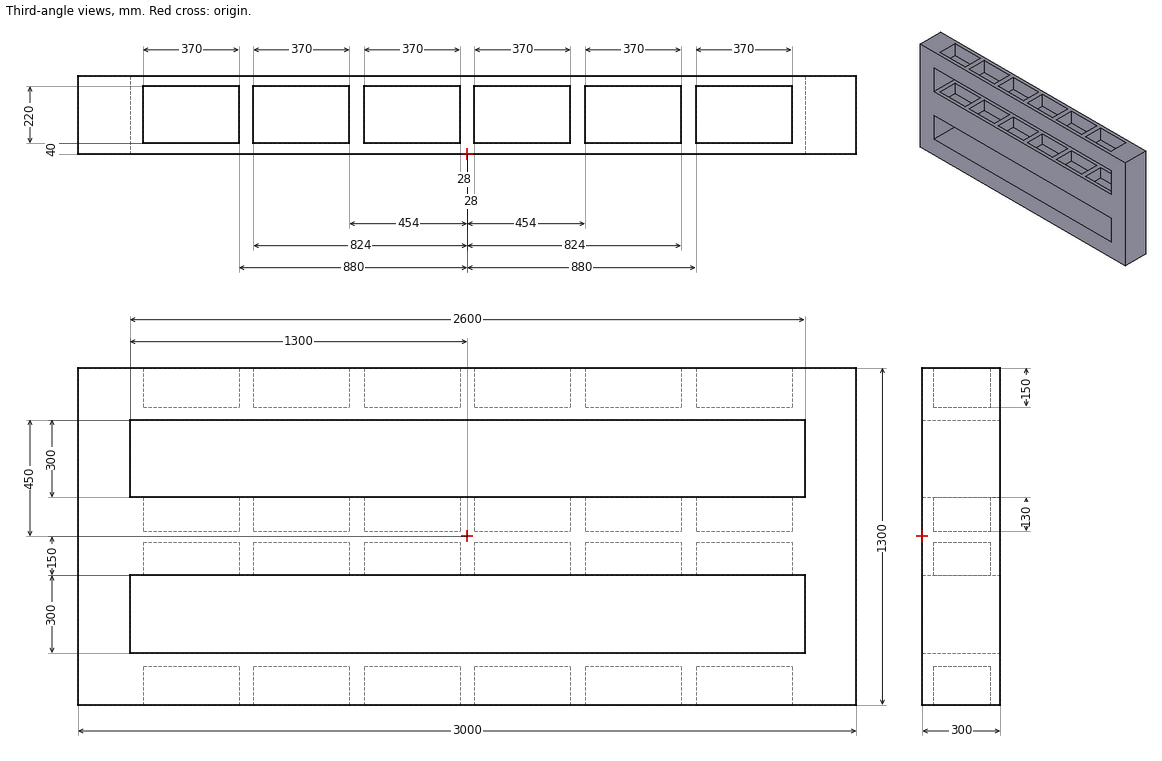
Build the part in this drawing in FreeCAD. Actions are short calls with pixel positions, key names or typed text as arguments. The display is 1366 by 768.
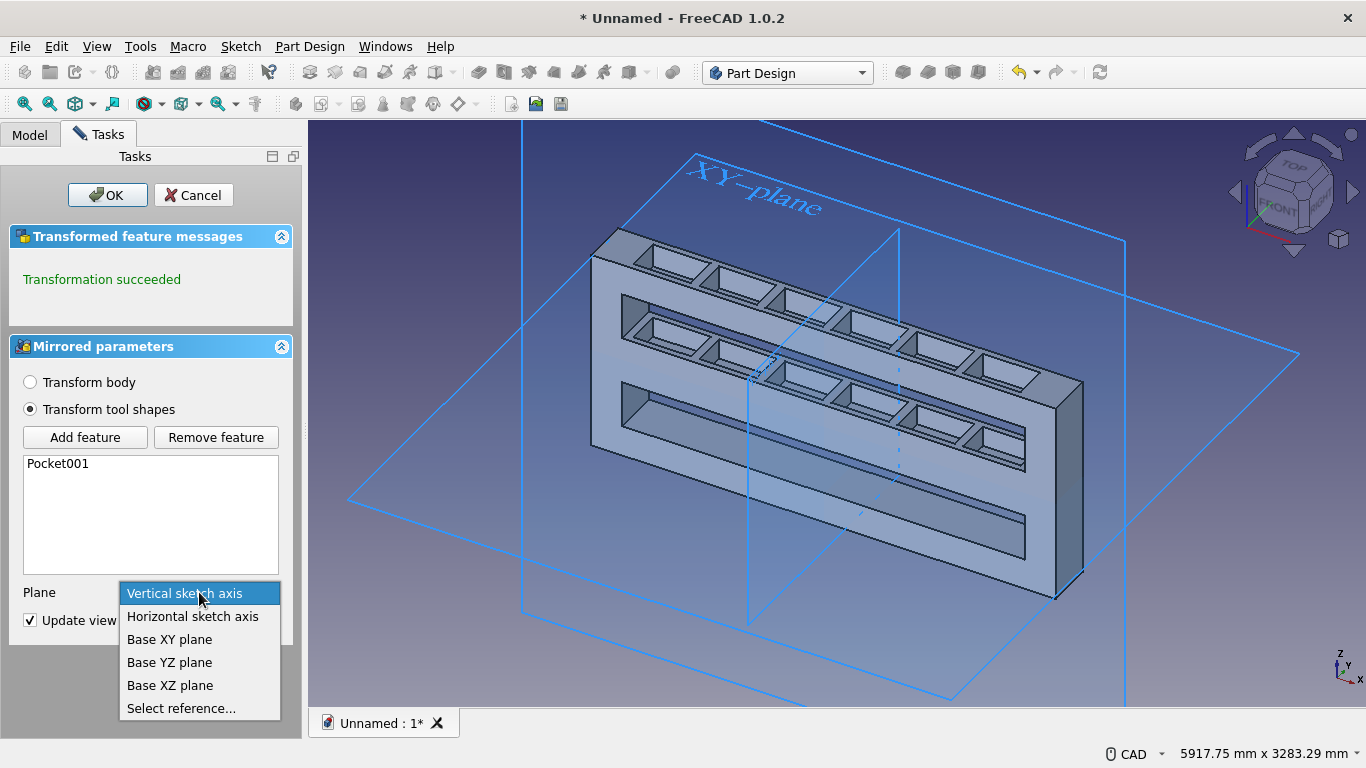
click(198, 640)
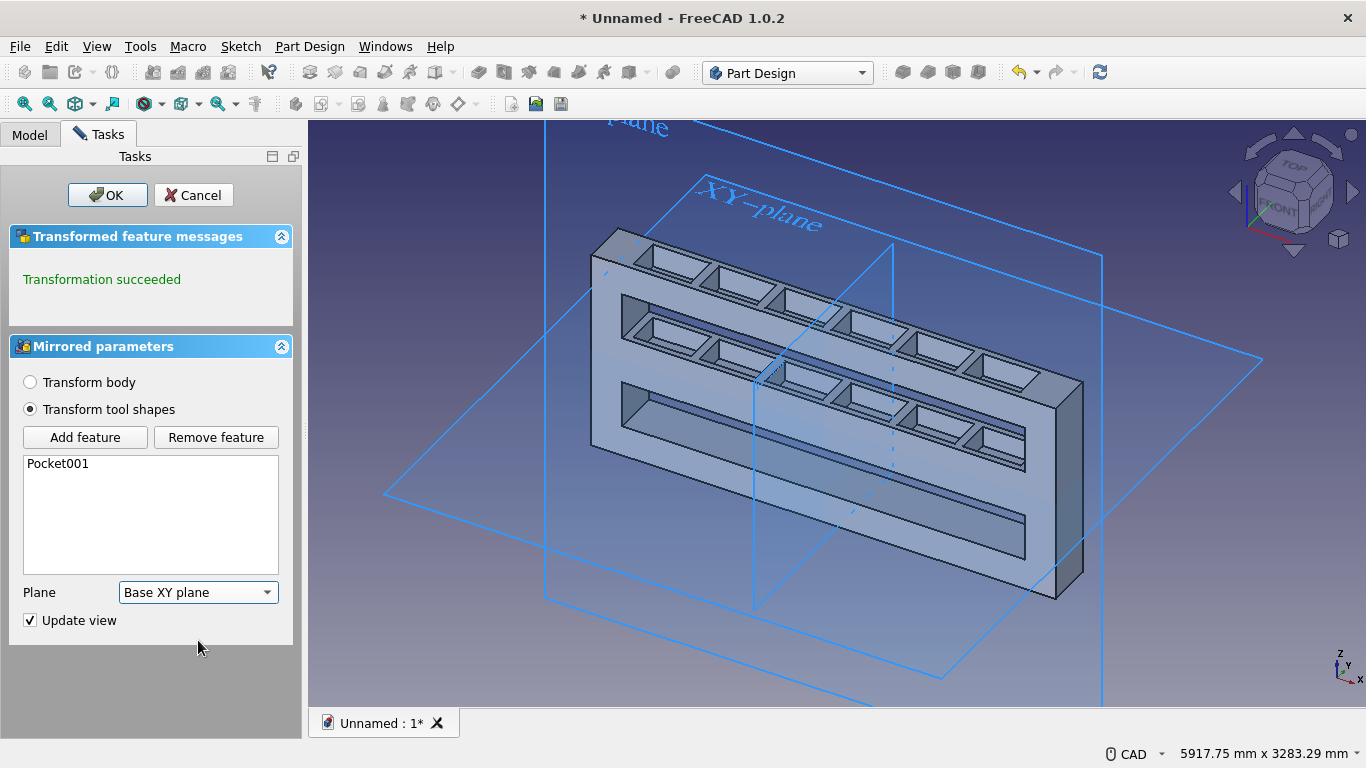
click(108, 195)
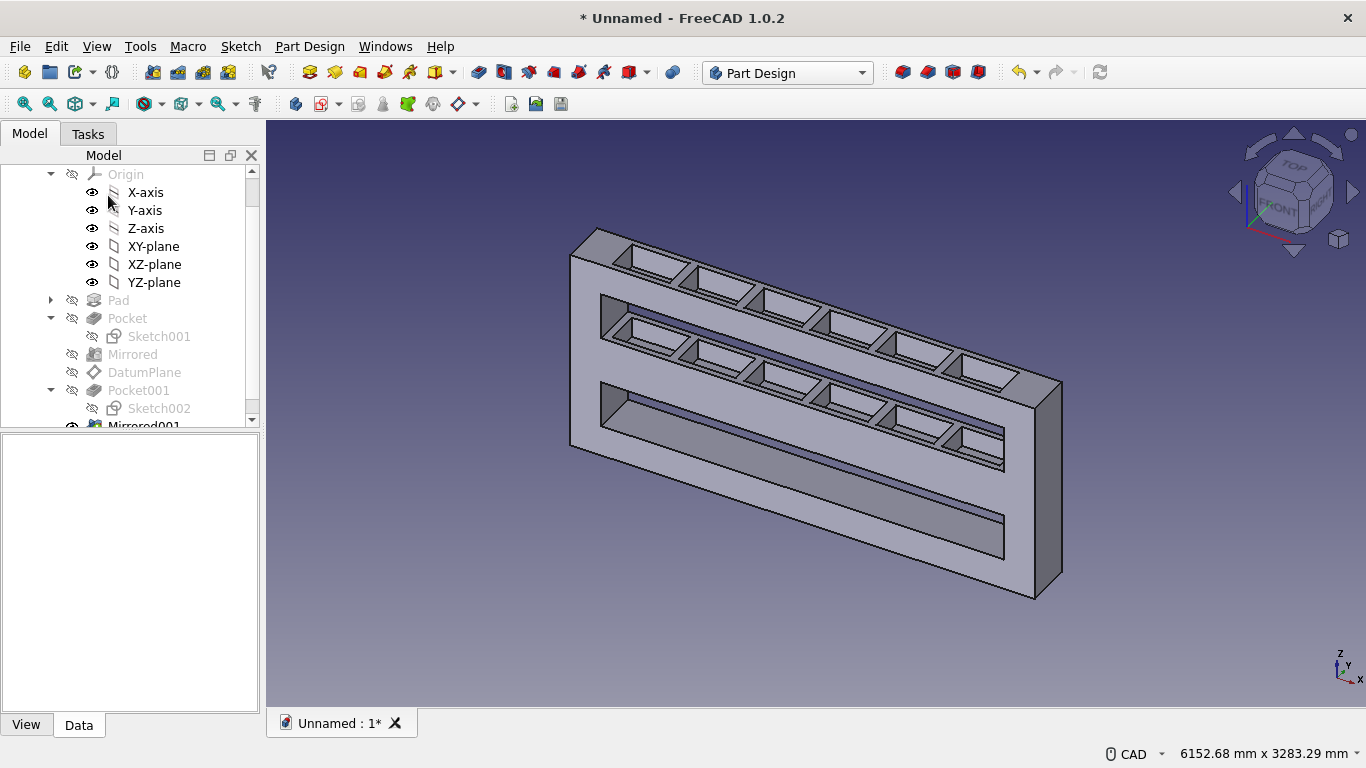
key(0)